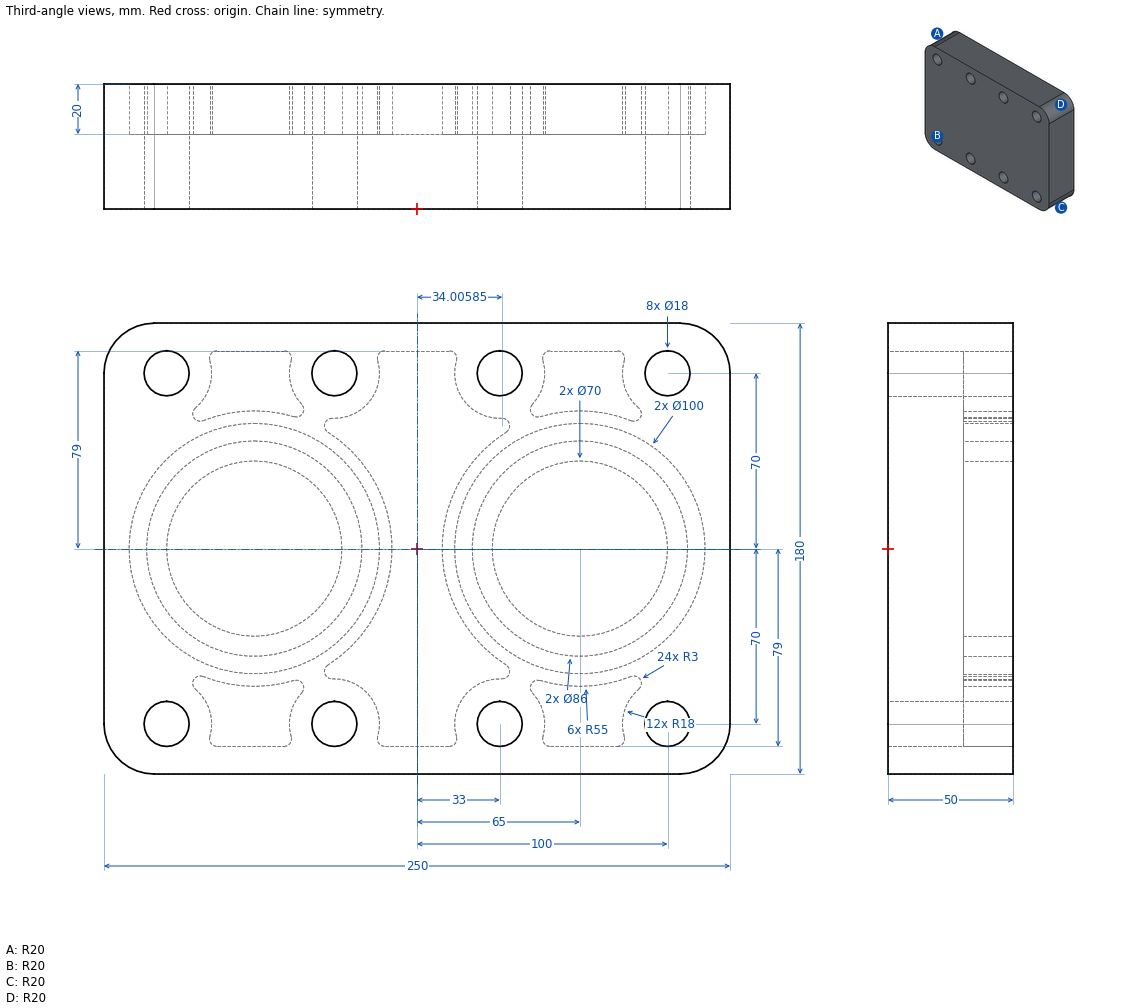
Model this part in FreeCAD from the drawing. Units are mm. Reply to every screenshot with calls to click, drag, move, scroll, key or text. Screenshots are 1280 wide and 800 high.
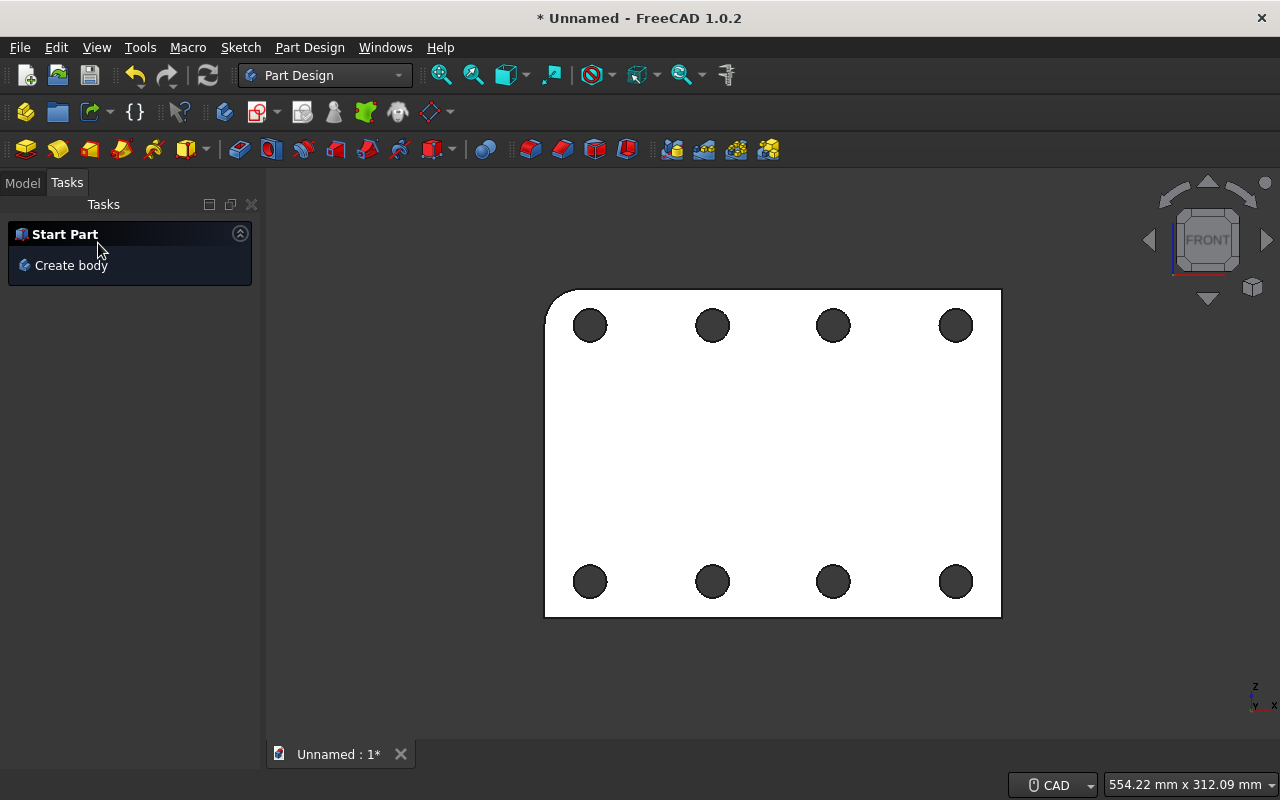
key(3)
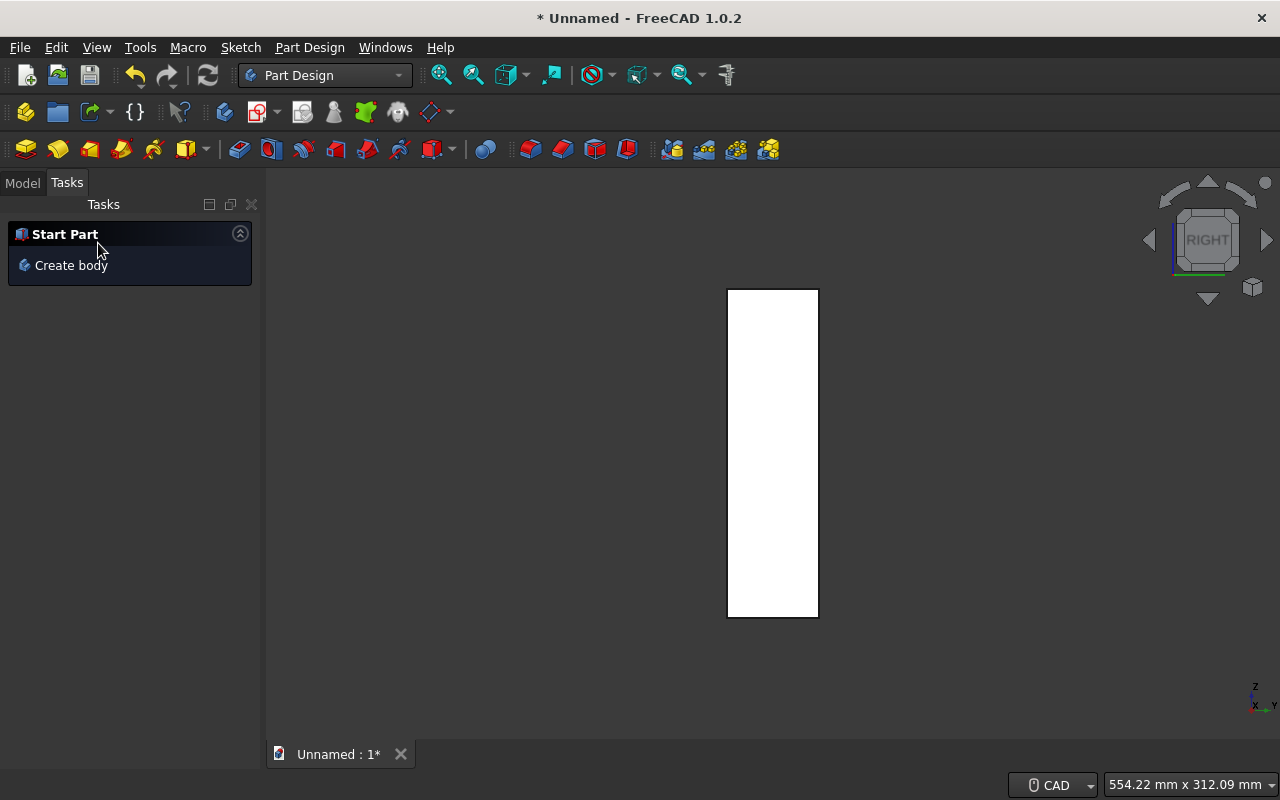
key(5)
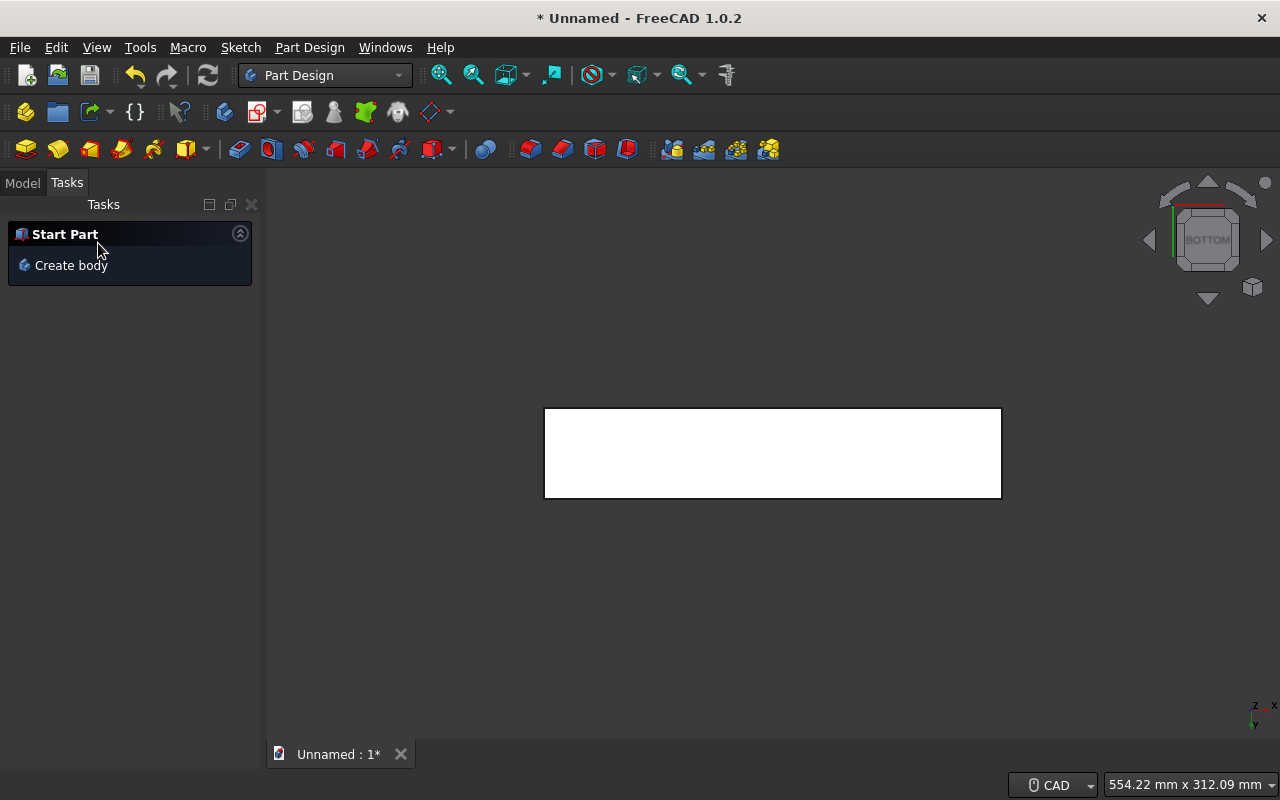
click(544, 452)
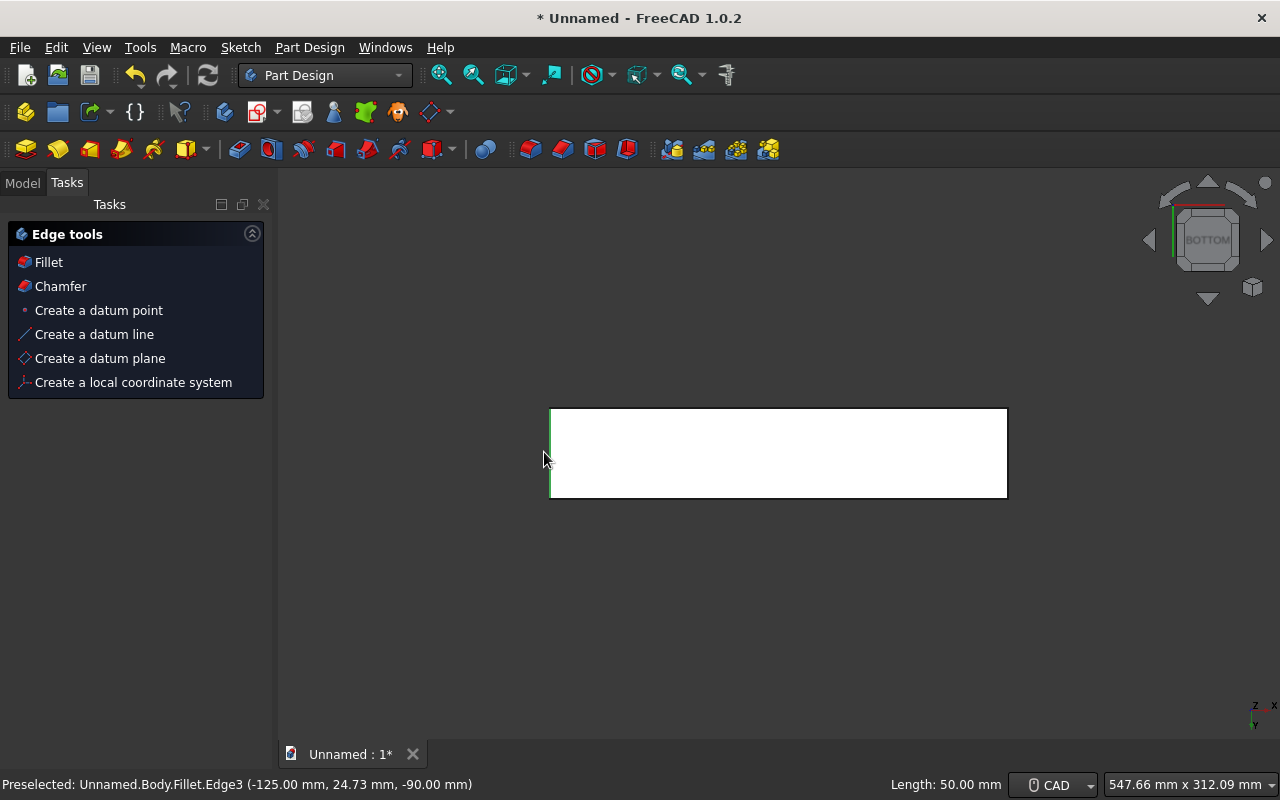
click(532, 150)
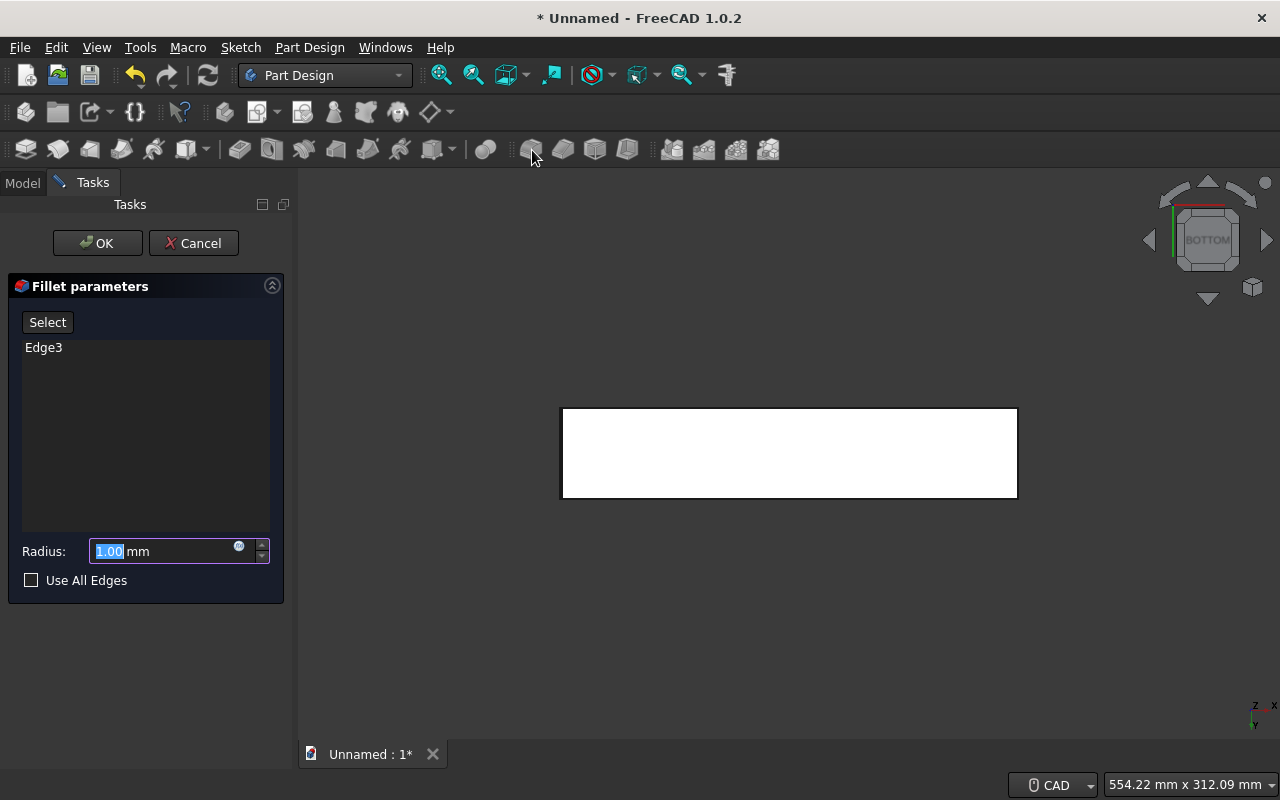
text(20)
key(Tab)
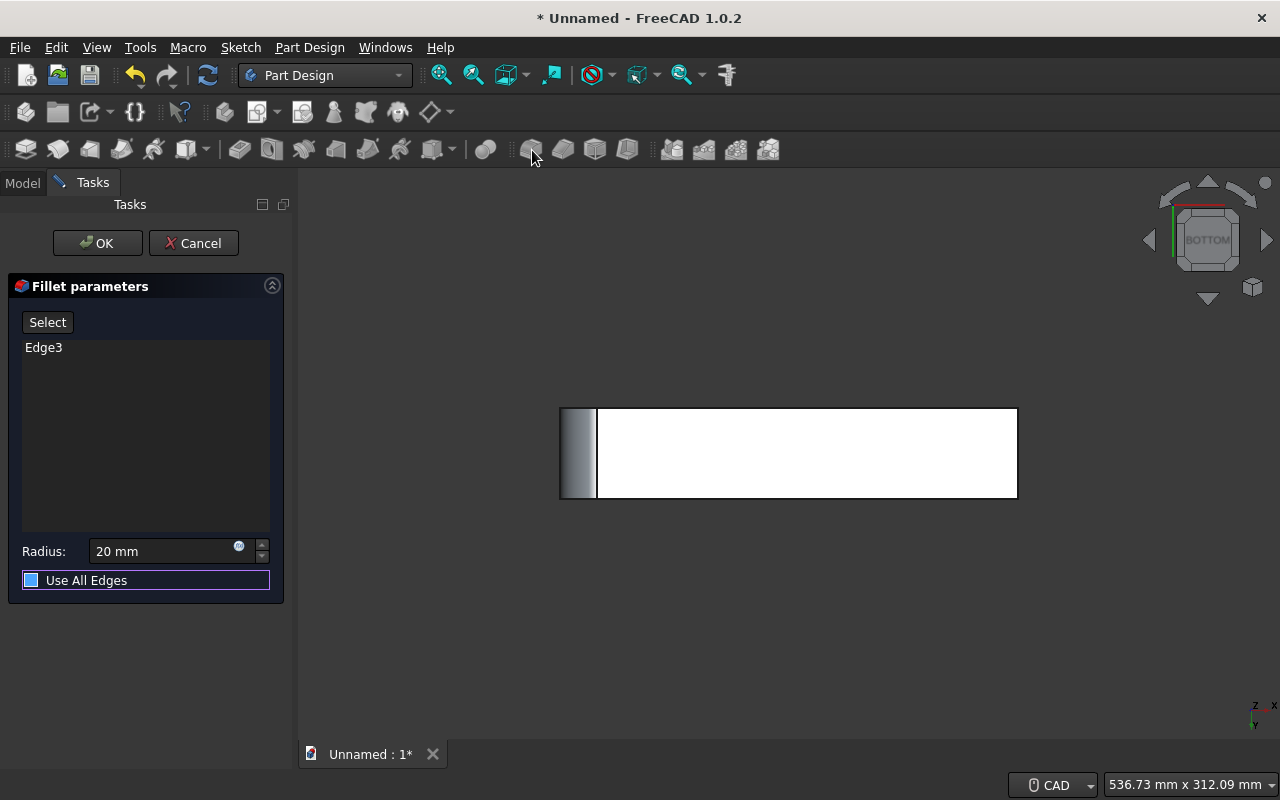
click(98, 243)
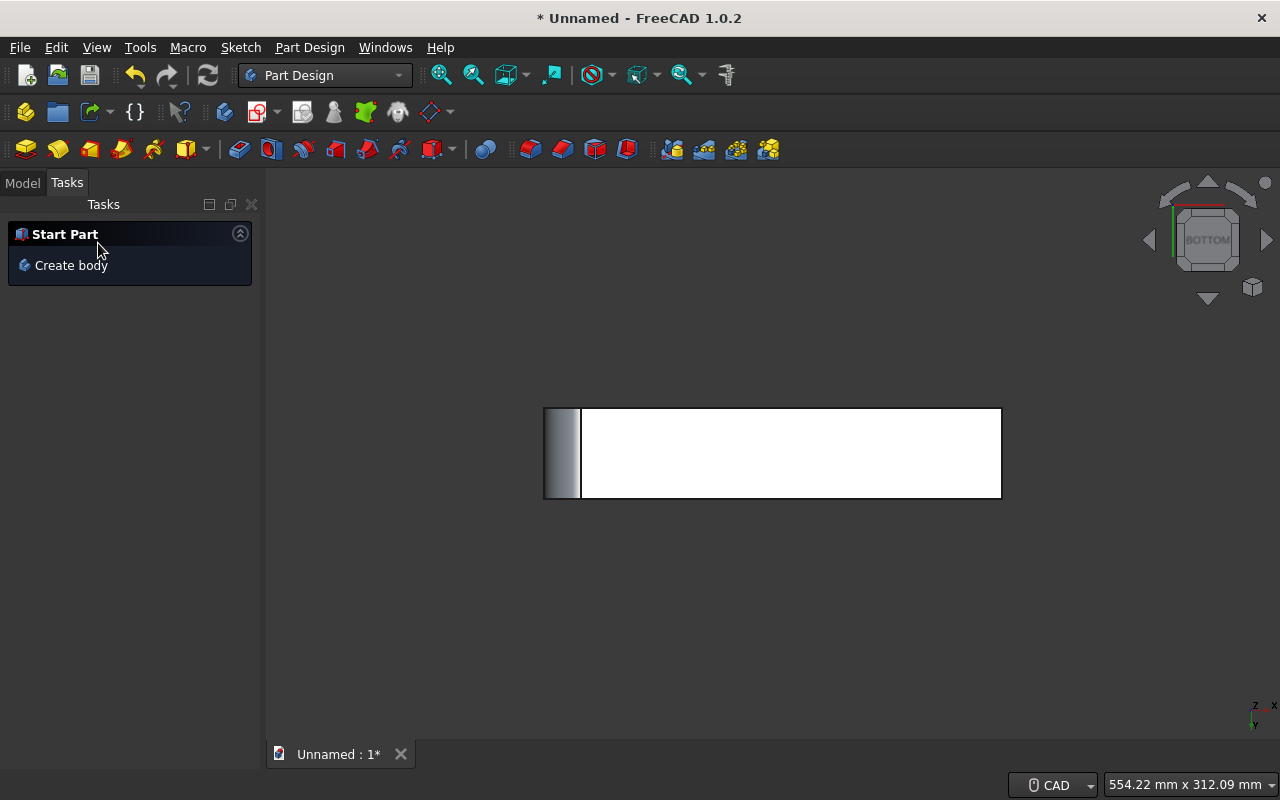
click(1002, 452)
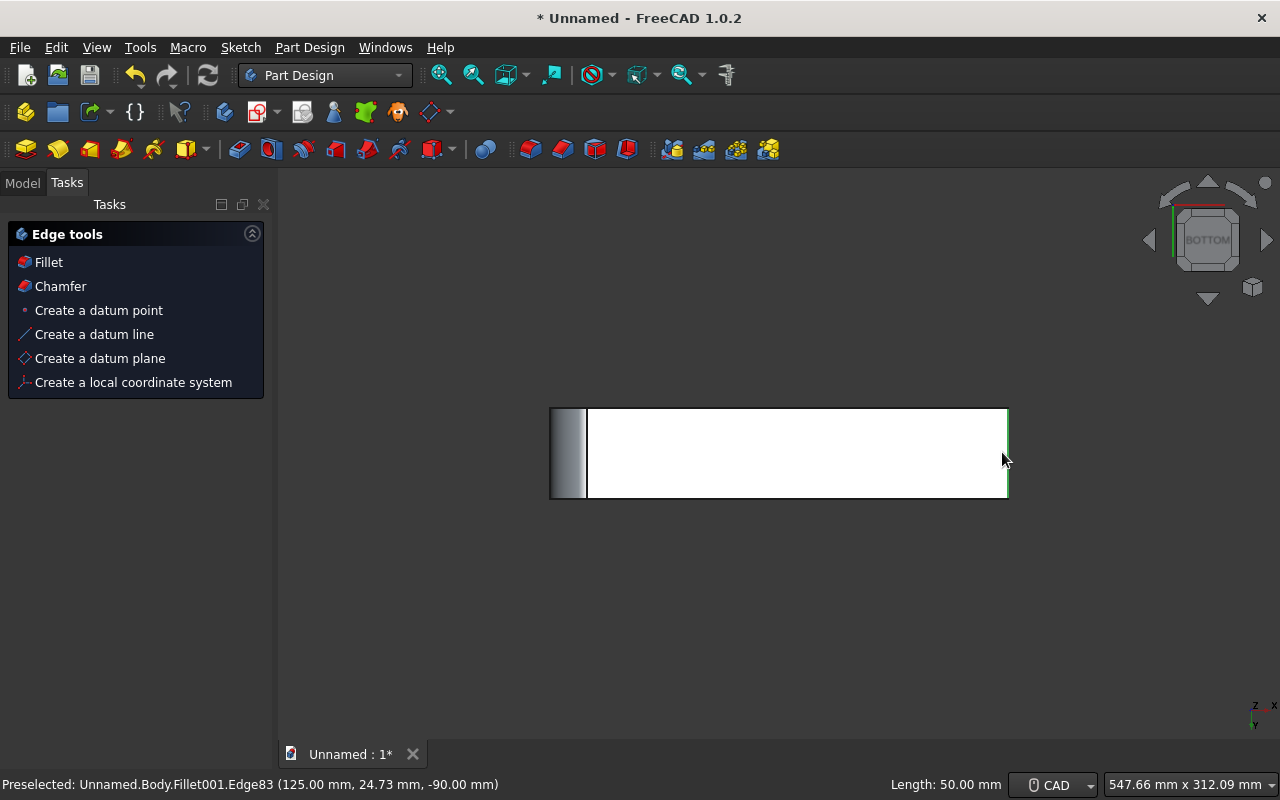
click(532, 150)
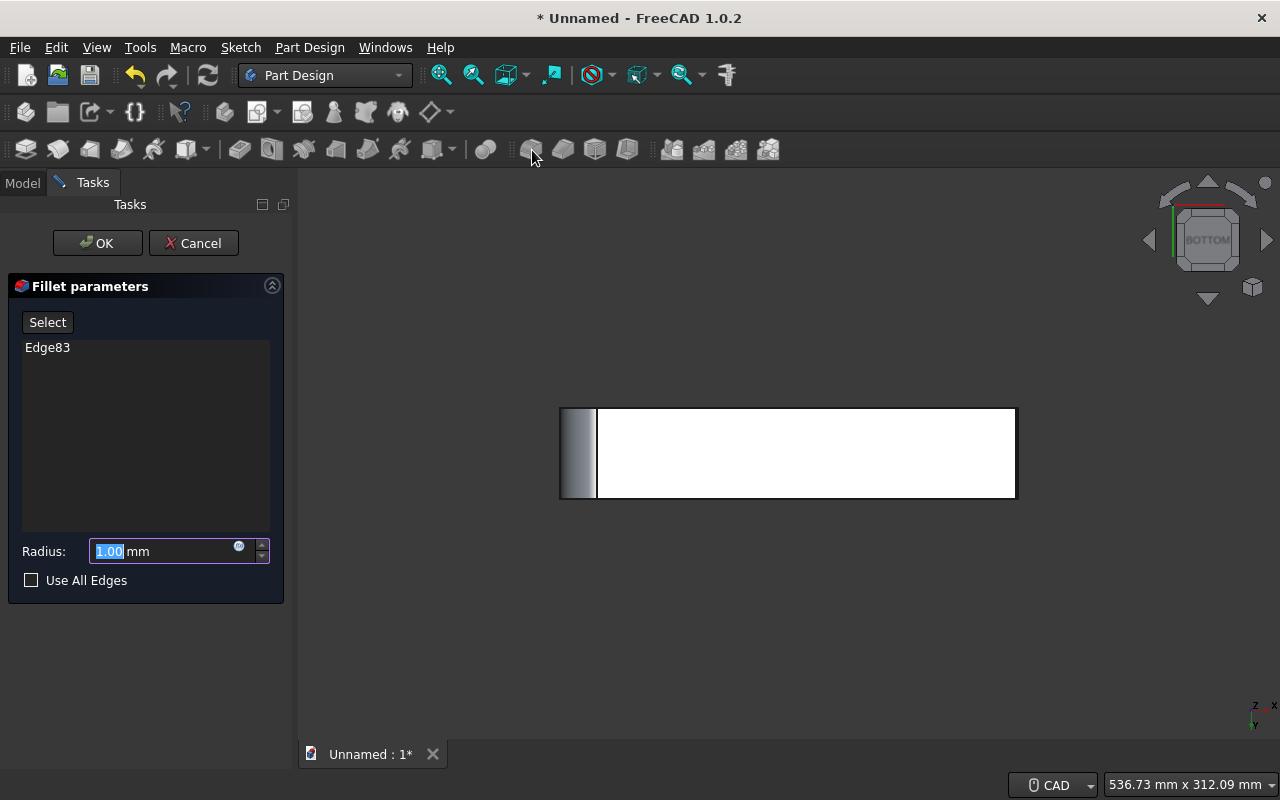
text(20)
key(Tab)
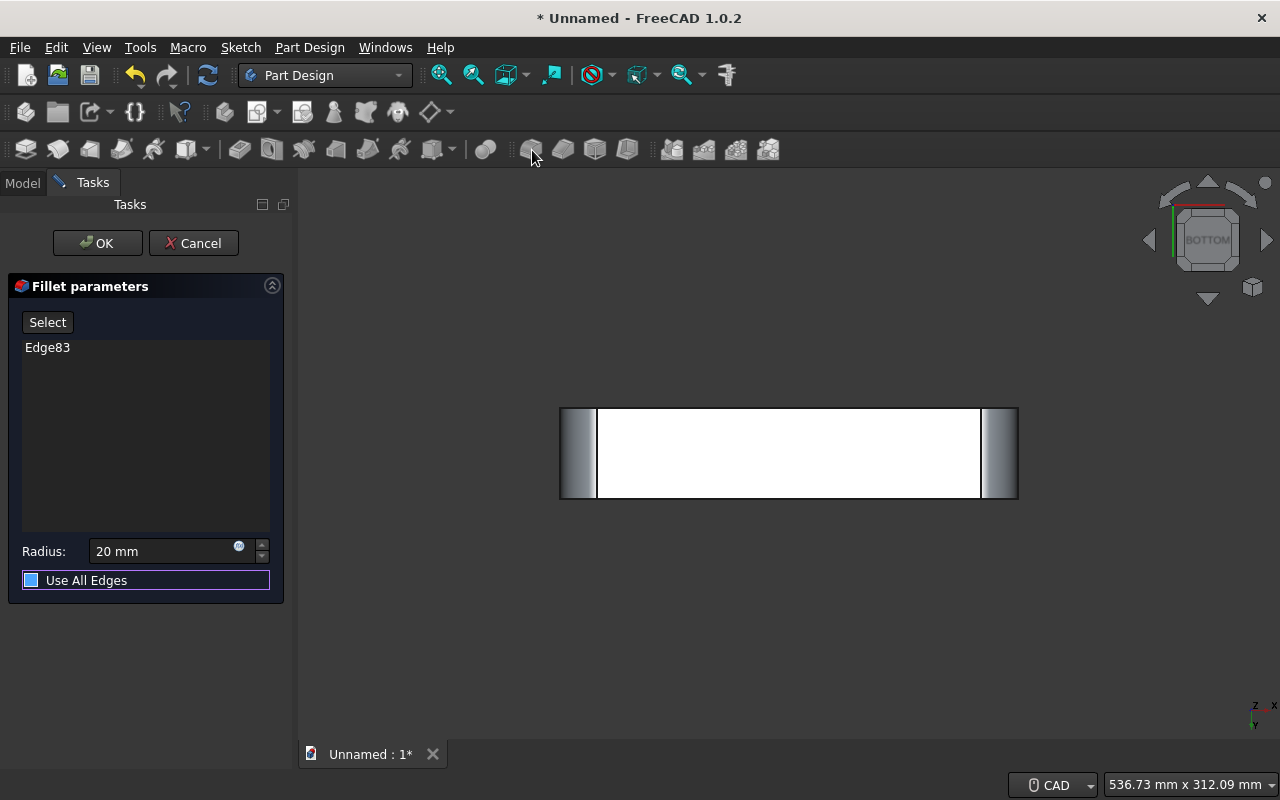
click(98, 243)